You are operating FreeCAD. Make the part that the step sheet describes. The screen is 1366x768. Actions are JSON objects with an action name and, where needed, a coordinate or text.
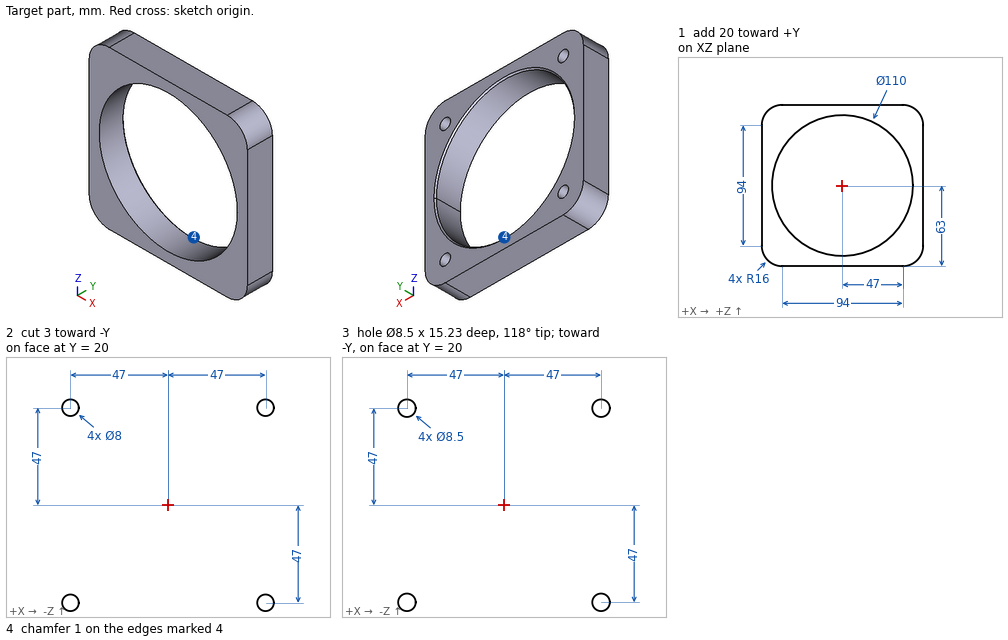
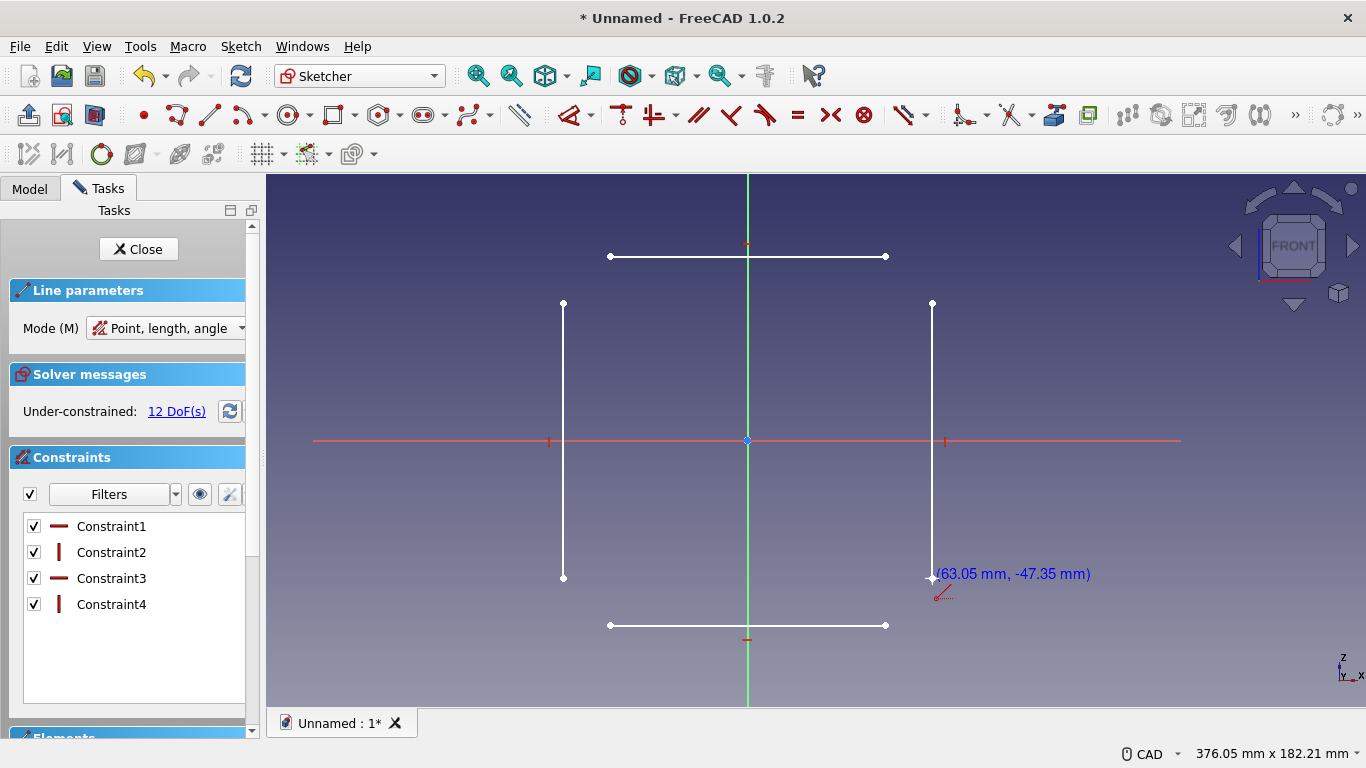
{"action": "key", "text": "g 3 a"}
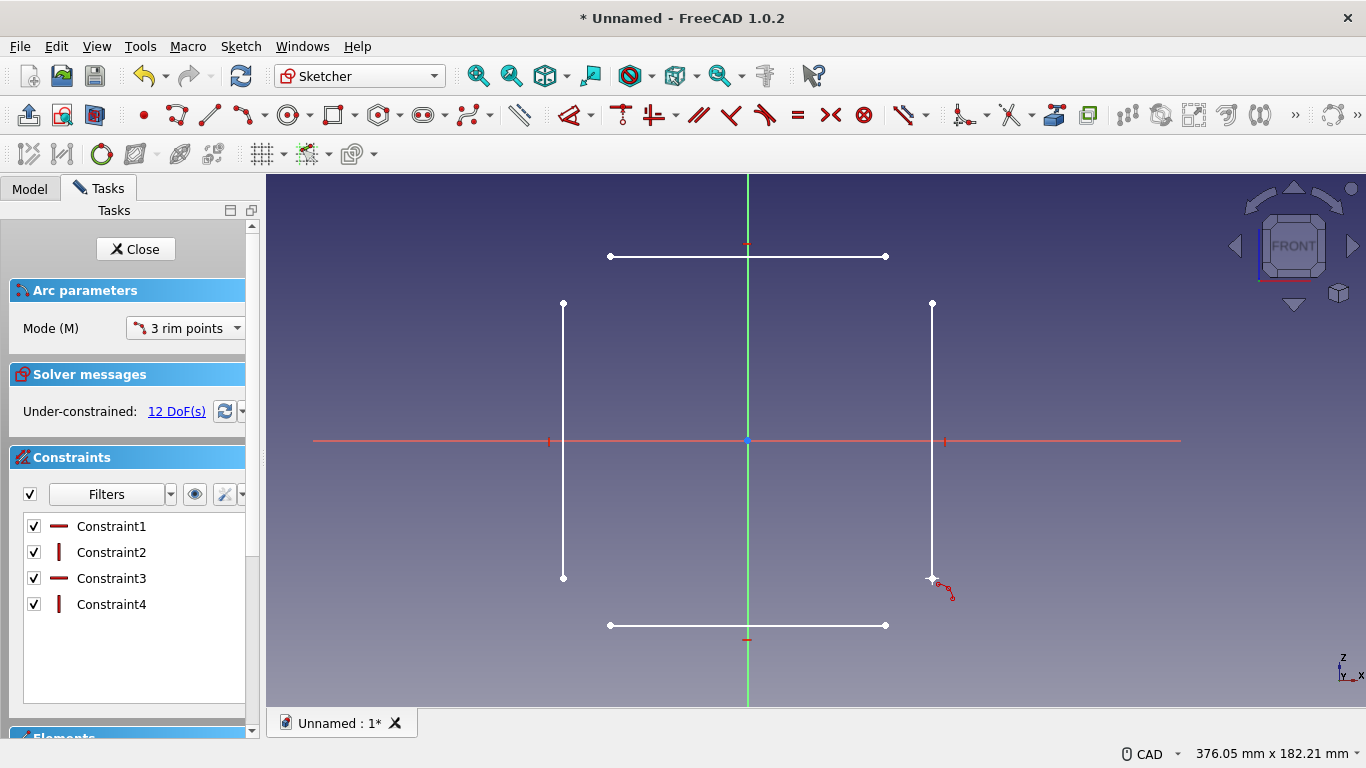
{"action": "left_click", "coordinate": [610, 626]}
{"action": "left_click", "coordinate": [563, 579]}
{"action": "left_click", "coordinate": [577, 611]}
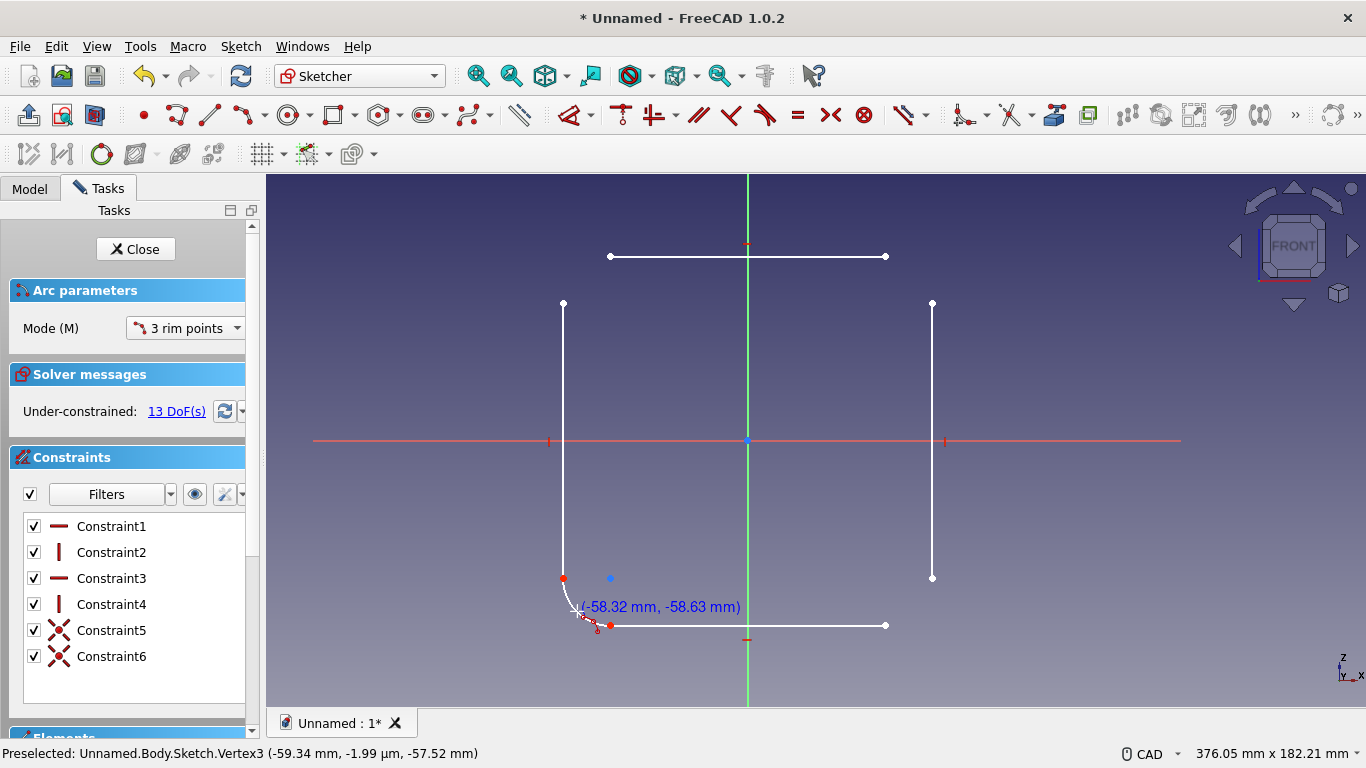
{"action": "left_click", "coordinate": [563, 304]}
{"action": "left_click", "coordinate": [610, 257]}
{"action": "left_click", "coordinate": [577, 270]}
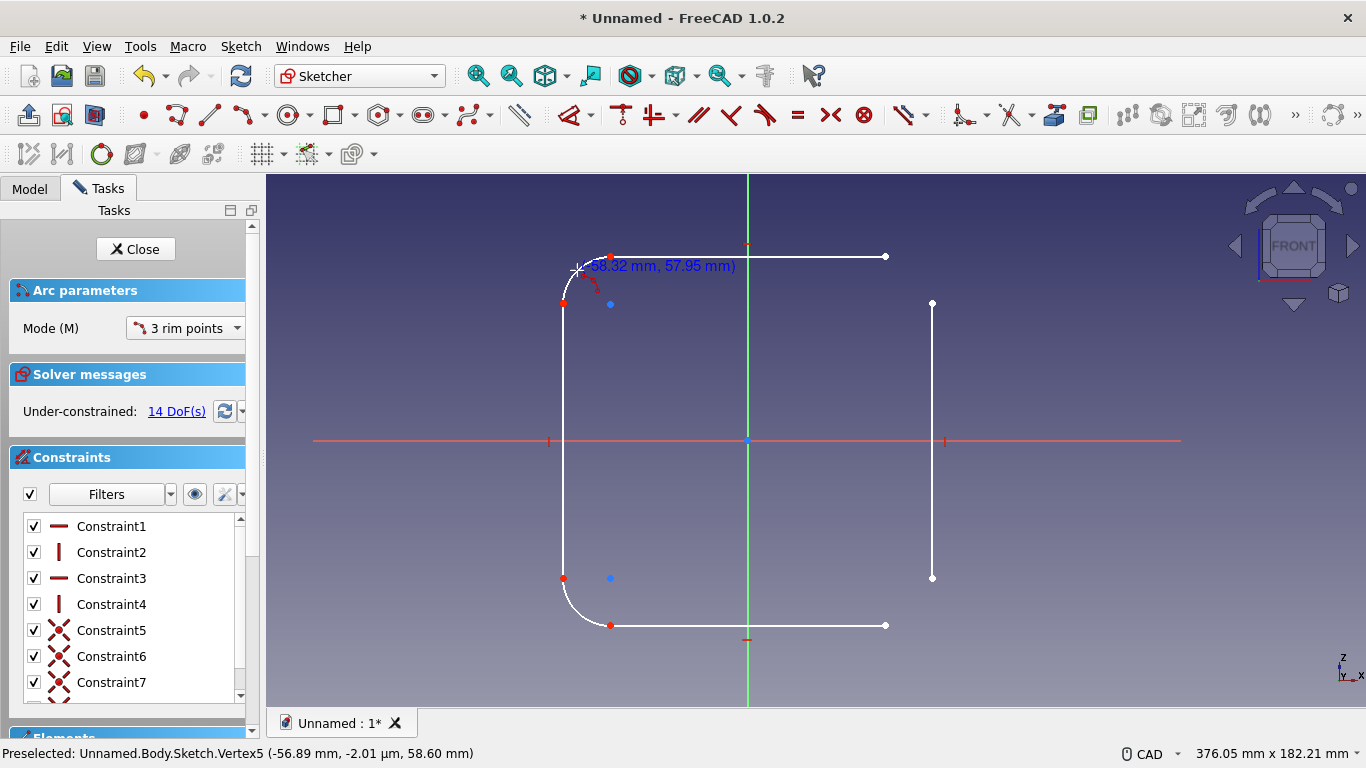
{"action": "left_click", "coordinate": [885, 257]}
{"action": "left_click", "coordinate": [932, 304]}
{"action": "left_click", "coordinate": [918, 270]}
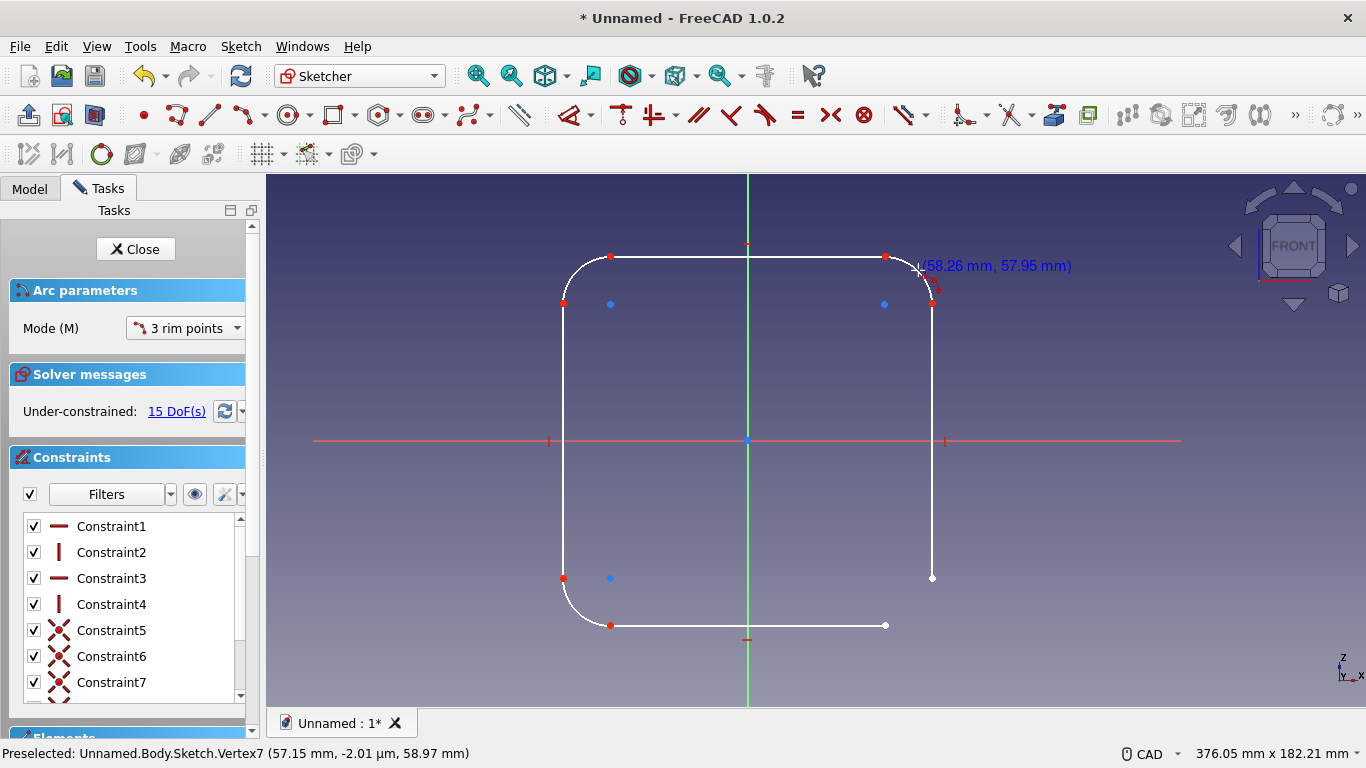
{"action": "left_click", "coordinate": [932, 579]}
{"action": "left_click", "coordinate": [885, 626]}
{"action": "left_click", "coordinate": [918, 611]}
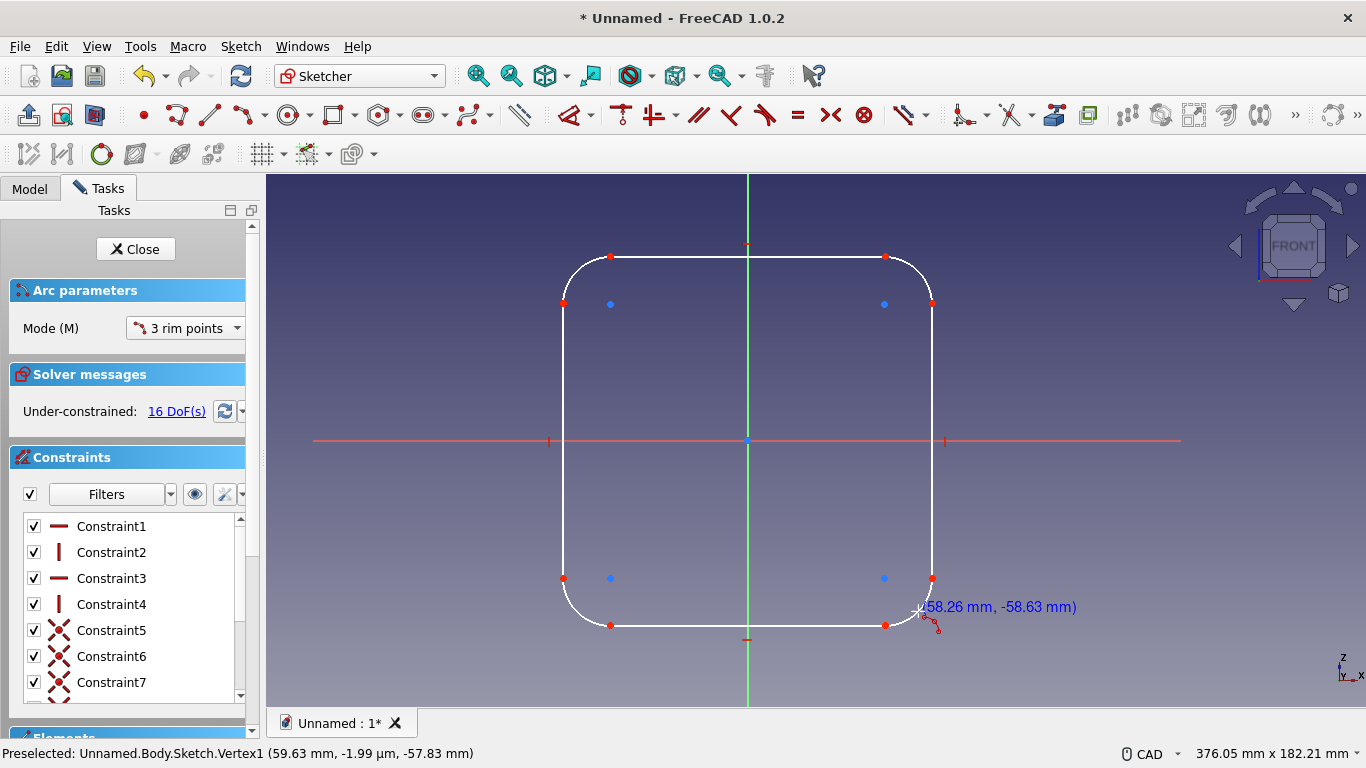
{"action": "left_click", "coordinate": [288, 116]}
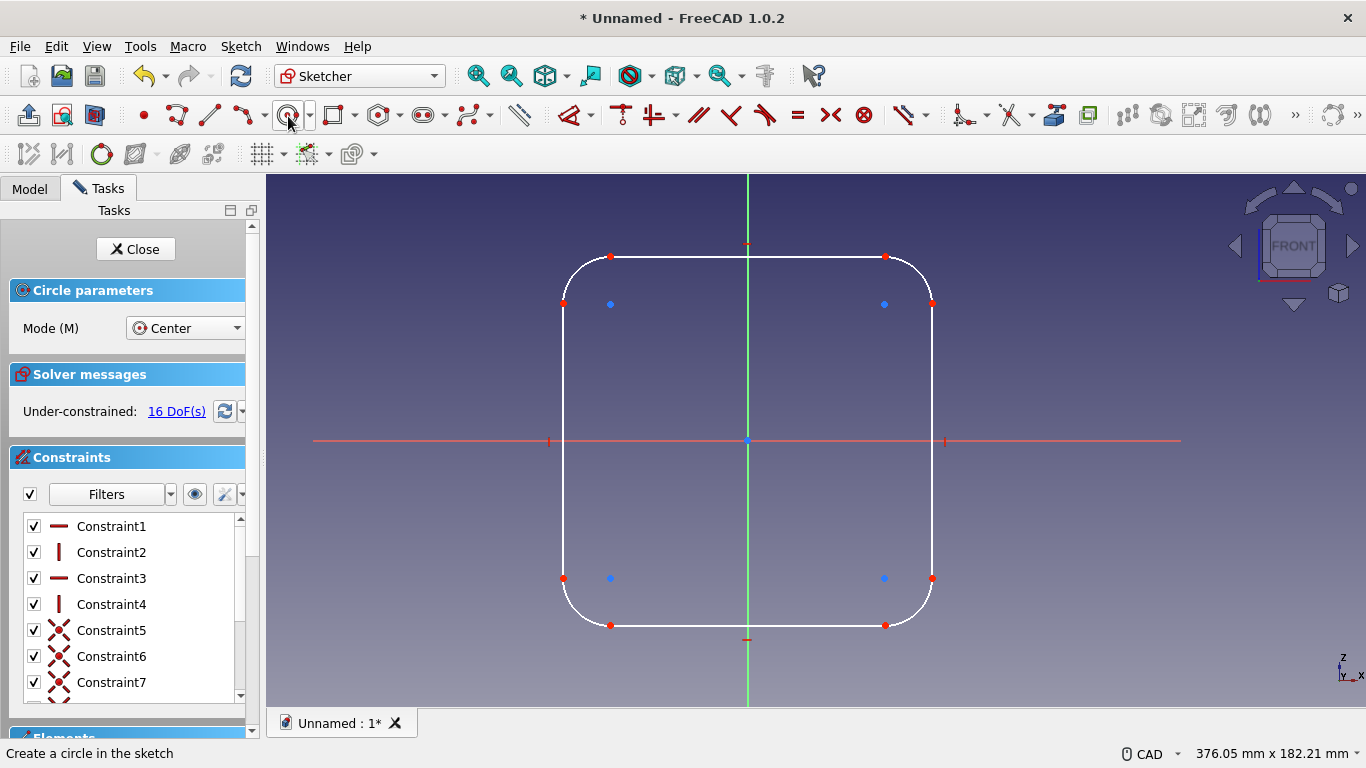
{"action": "left_click", "coordinate": [748, 440]}
{"action": "left_click", "coordinate": [861, 327]}
{"action": "key", "text": "Escape"}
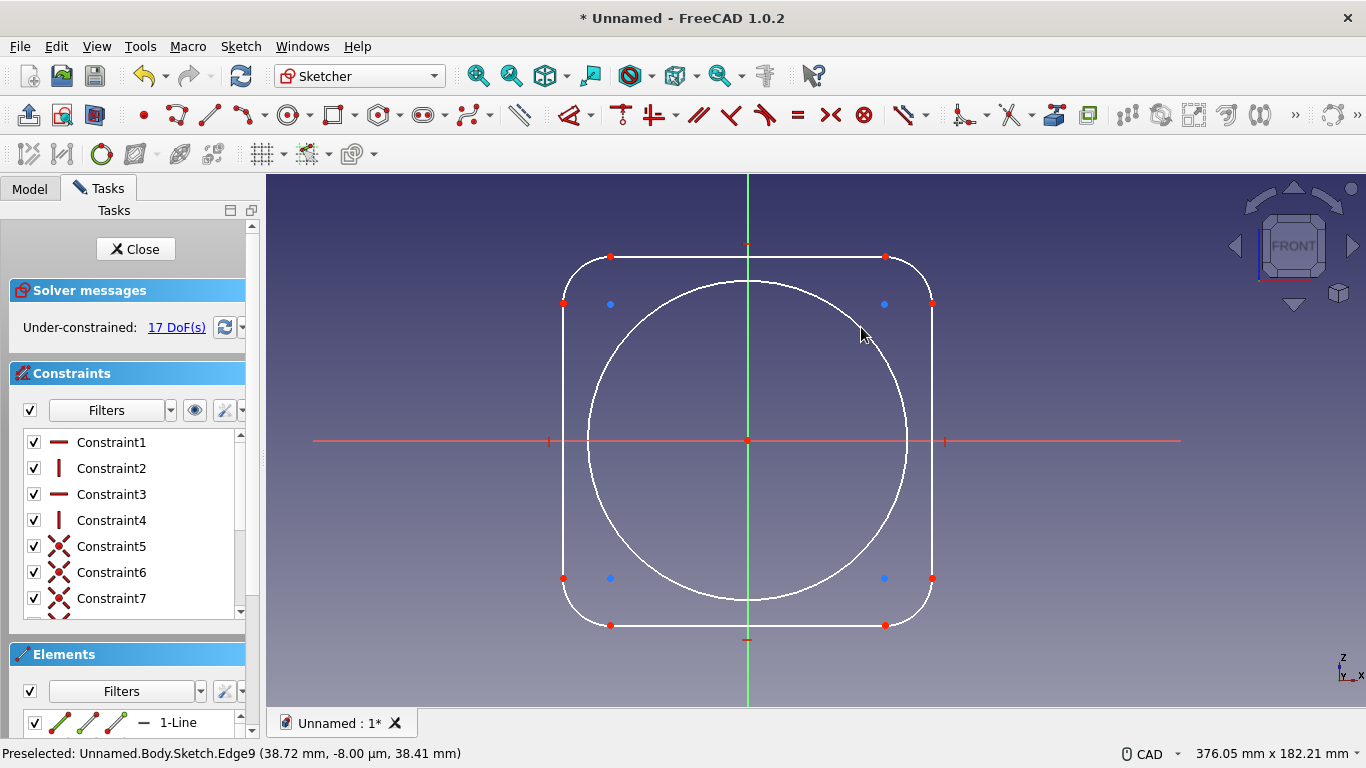
{"action": "left_click", "coordinate": [802, 626]}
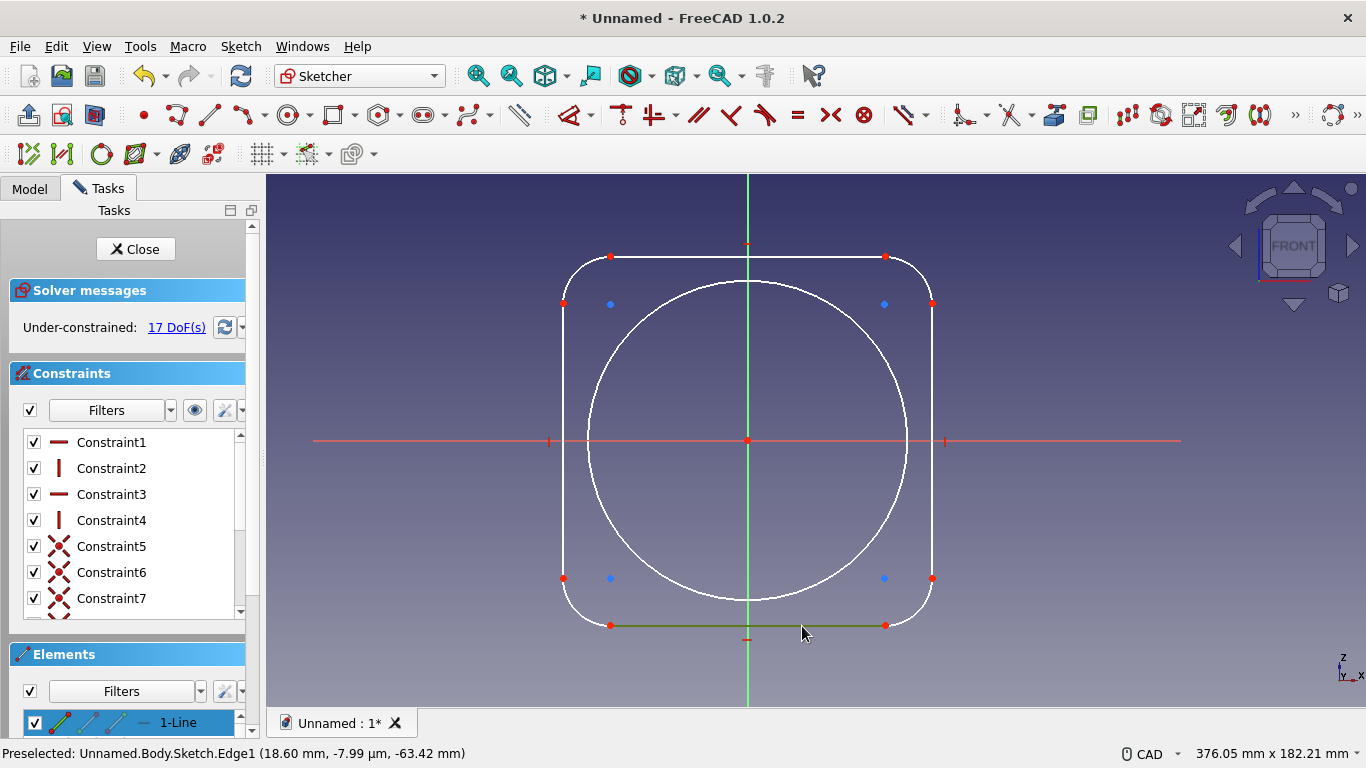
{"action": "left_click", "coordinate": [568, 600]}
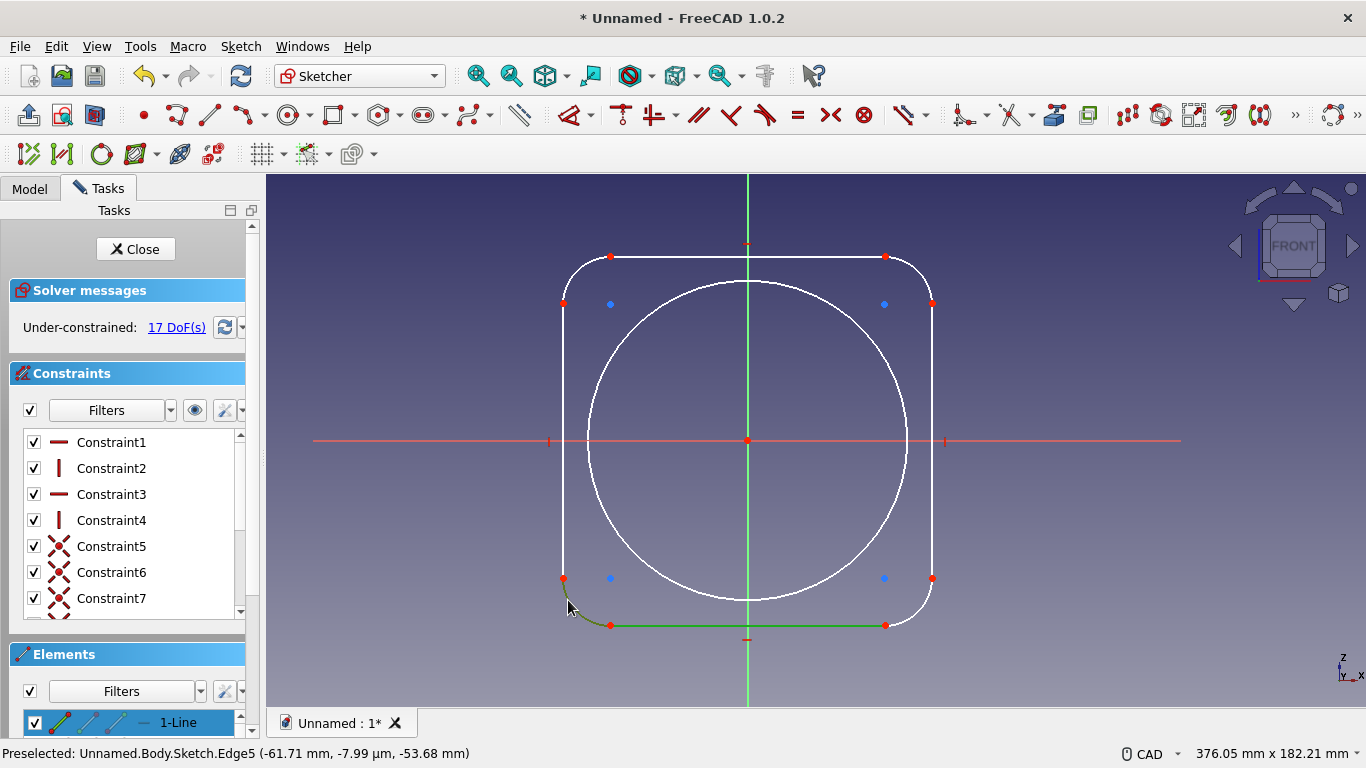
{"action": "key", "text": "t"}